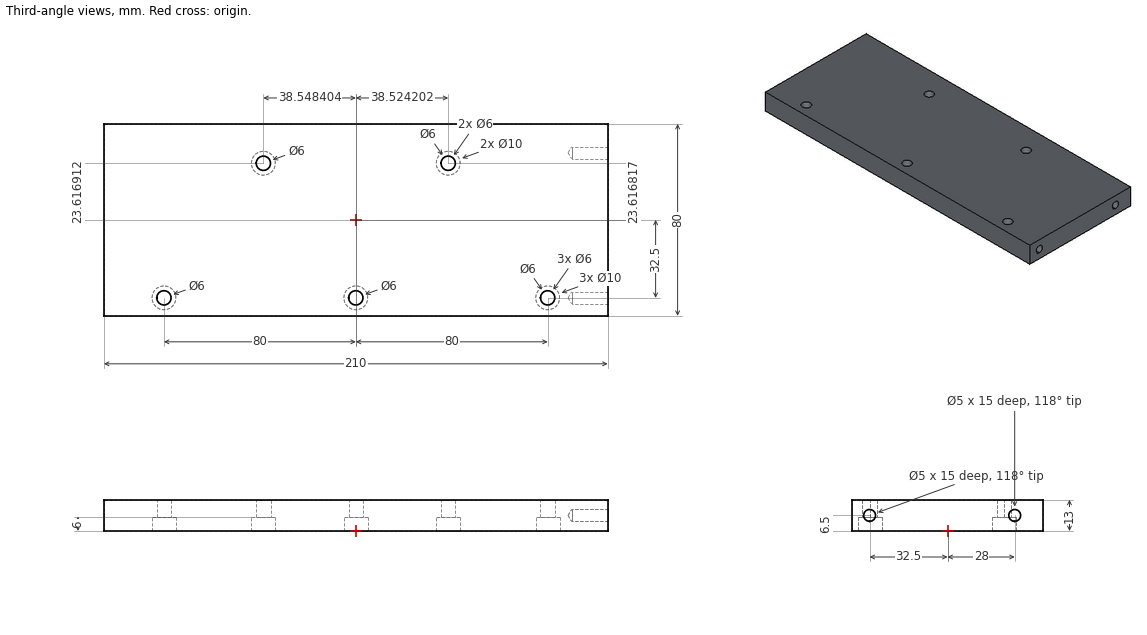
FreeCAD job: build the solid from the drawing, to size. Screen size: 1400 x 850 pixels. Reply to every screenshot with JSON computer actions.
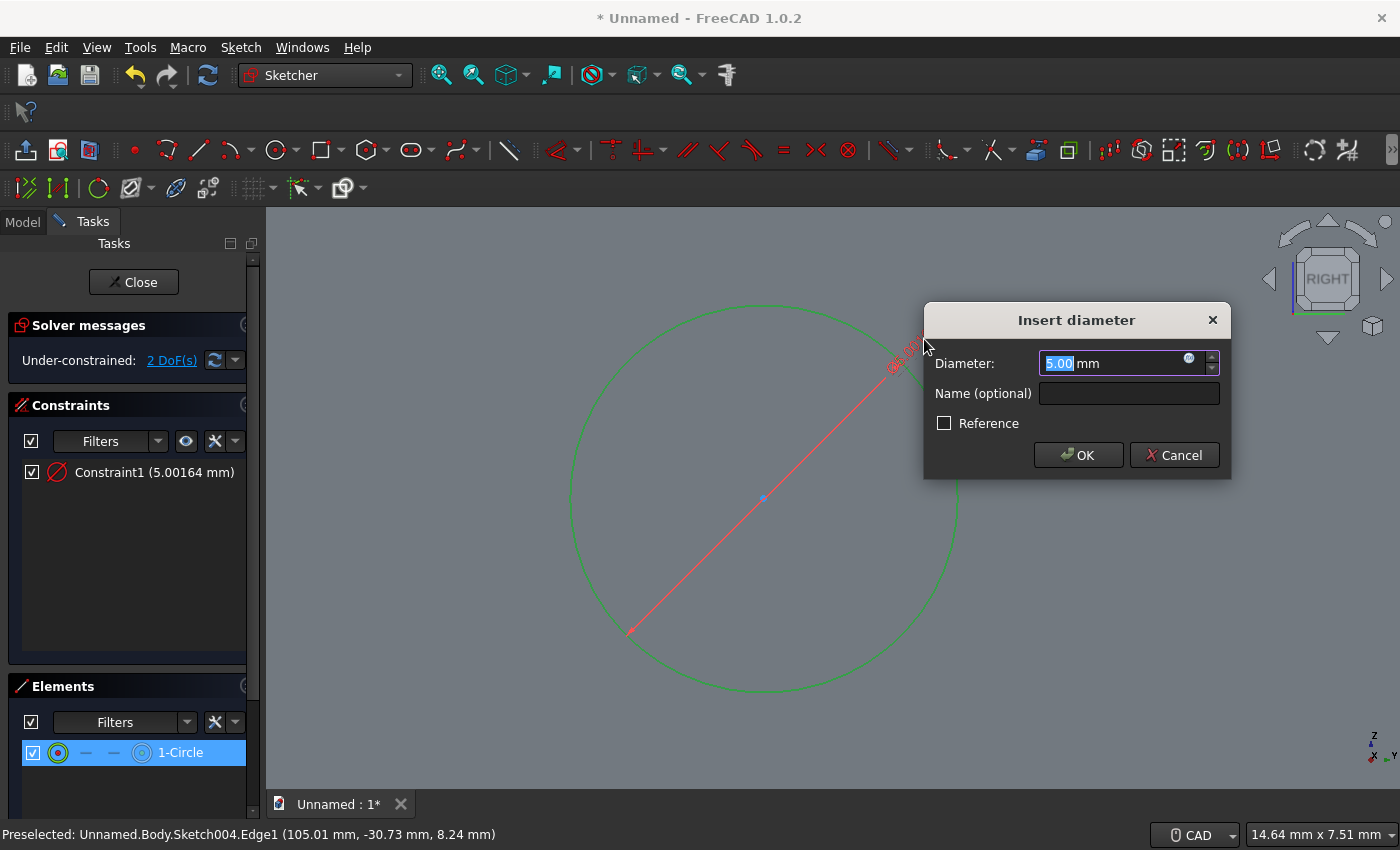
{"action": "type", "text": "5"}
{"action": "key", "text": "Return"}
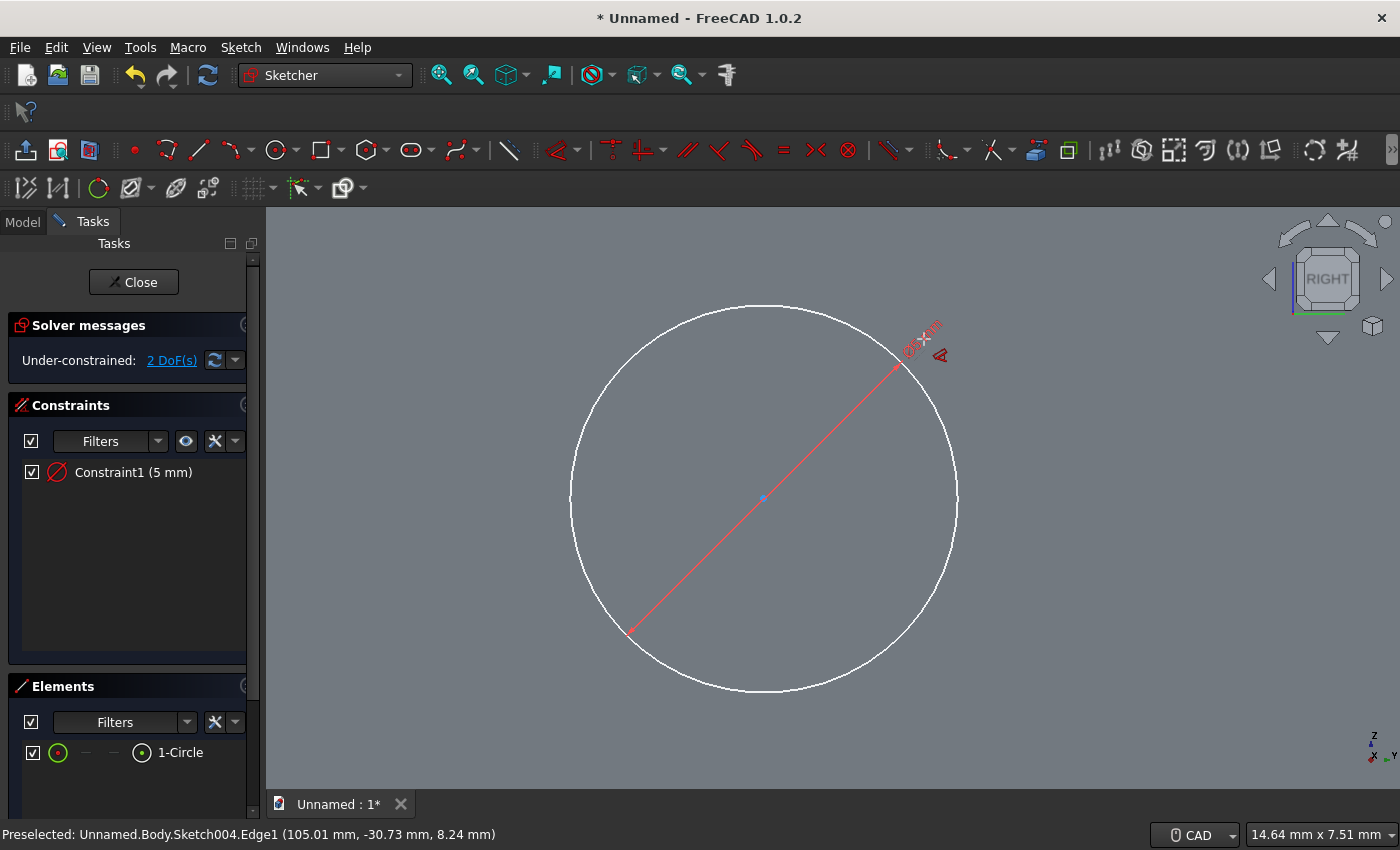
{"action": "left_click", "coordinate": [764, 499]}
{"action": "left_click", "coordinate": [730, 630]}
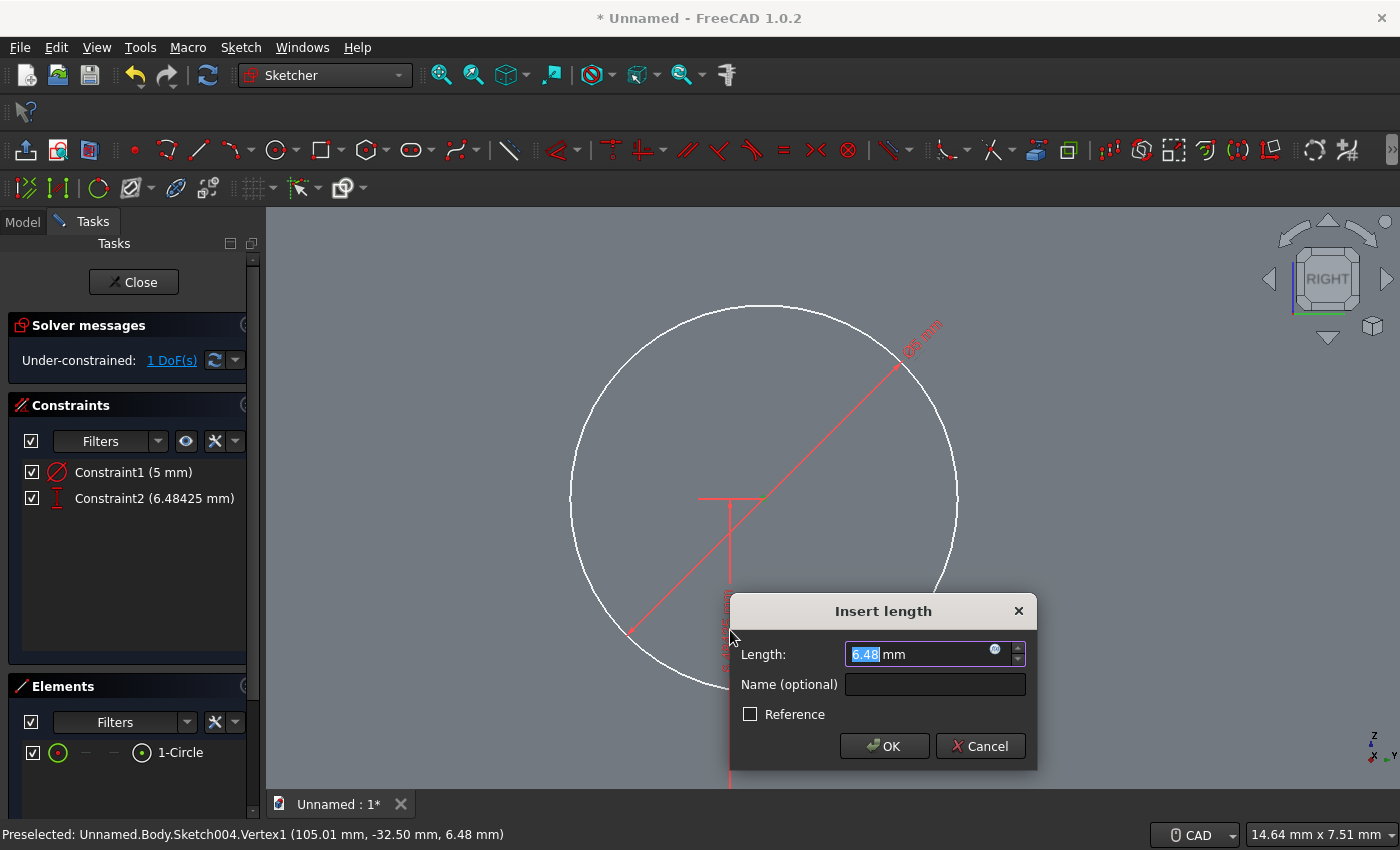
{"action": "type", "text": "6.5"}
{"action": "key", "text": "Return"}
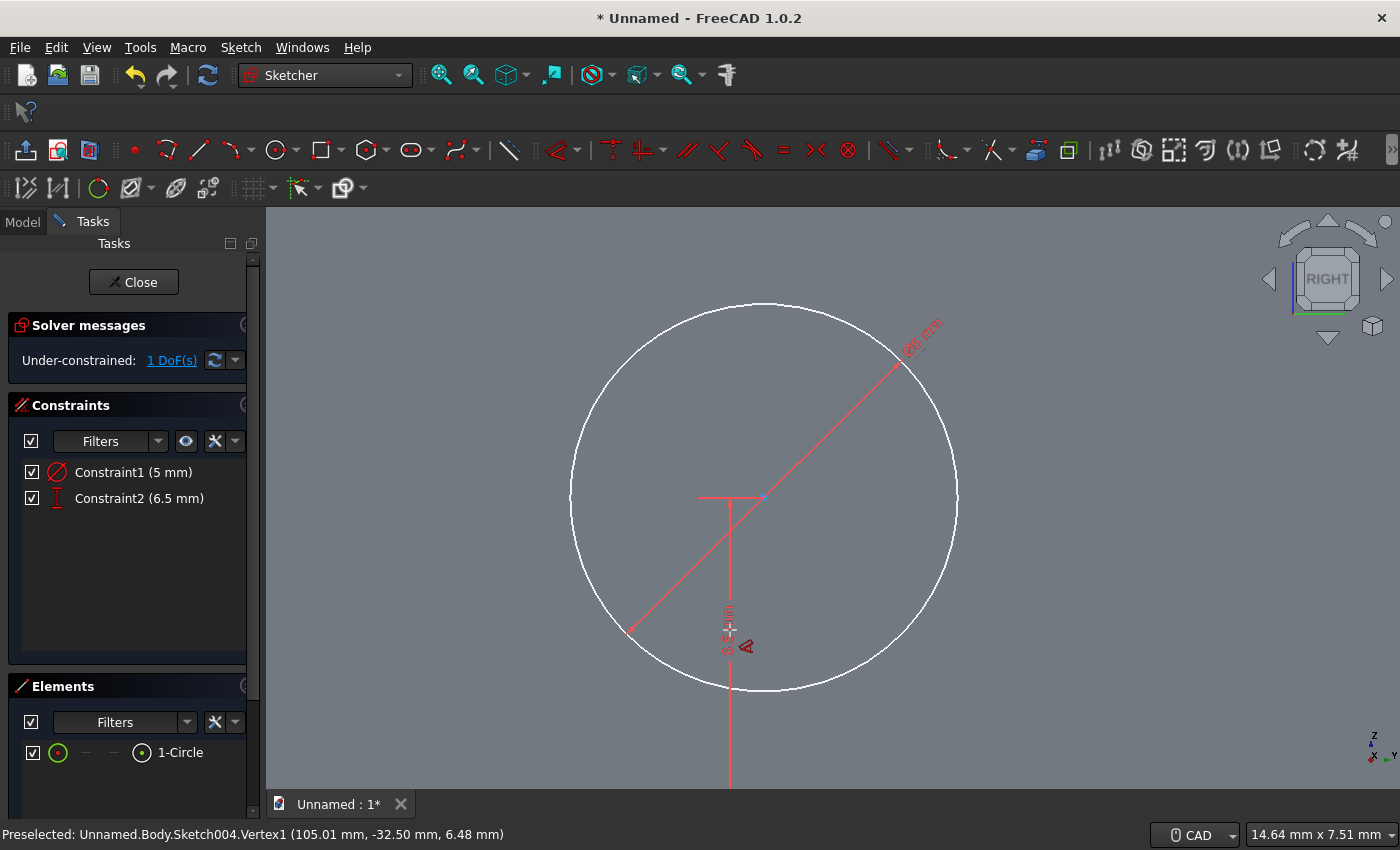
{"action": "left_click", "coordinate": [764, 498]}
{"action": "left_click", "coordinate": [999, 464]}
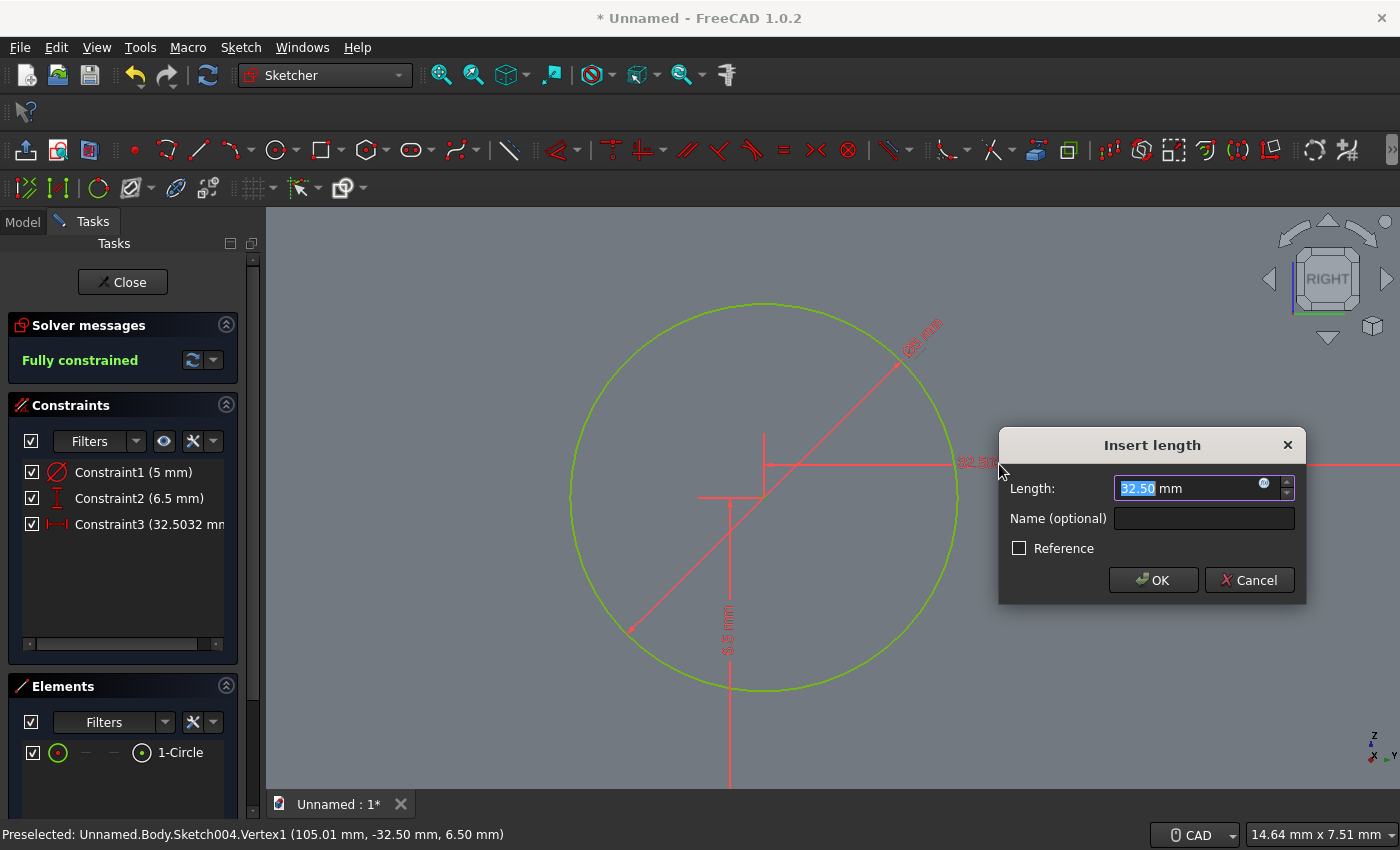
{"action": "type", "text": "32.5"}
{"action": "key", "text": "Return"}
{"action": "key", "text": "Escape"}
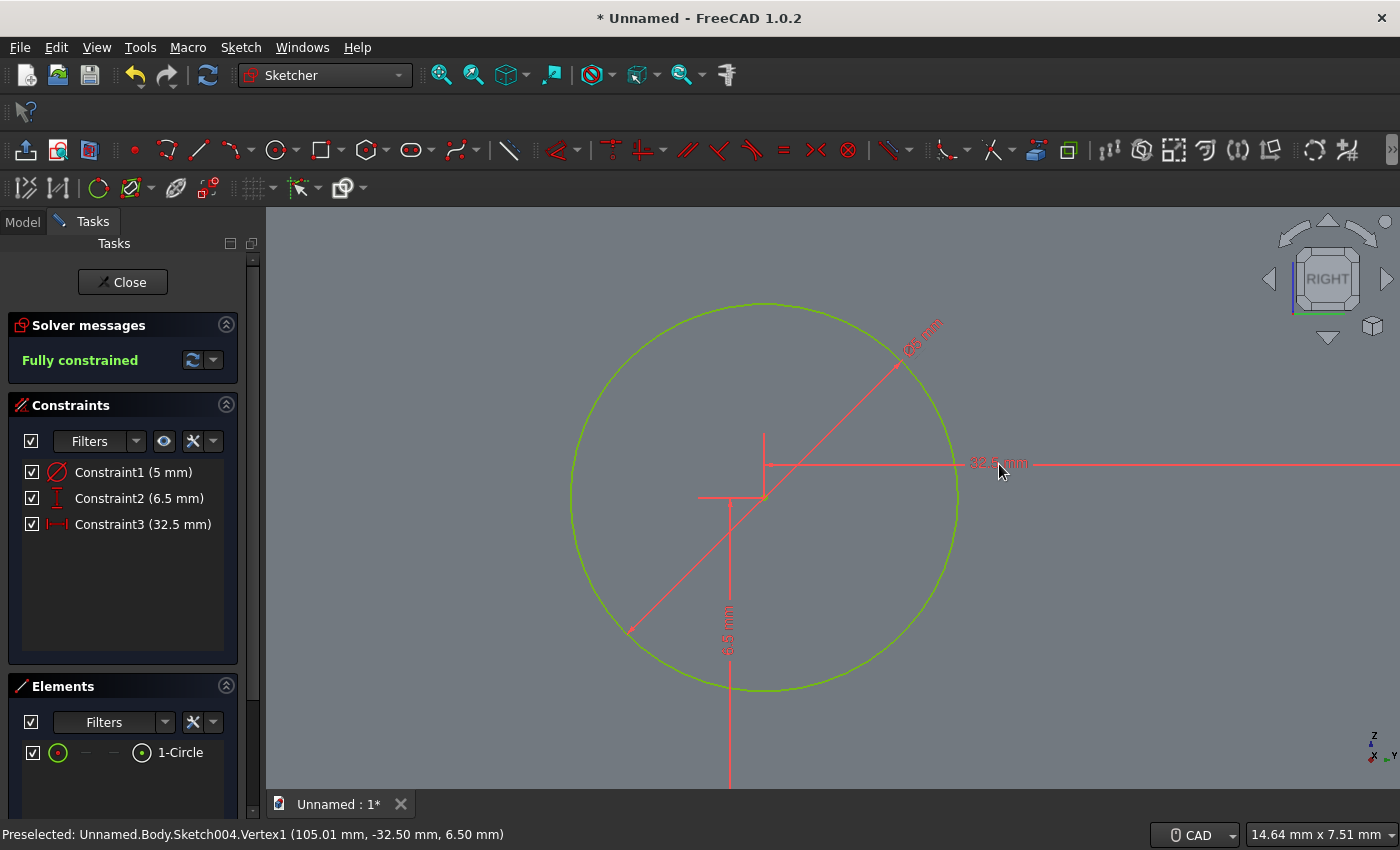
{"action": "left_click", "coordinate": [123, 282]}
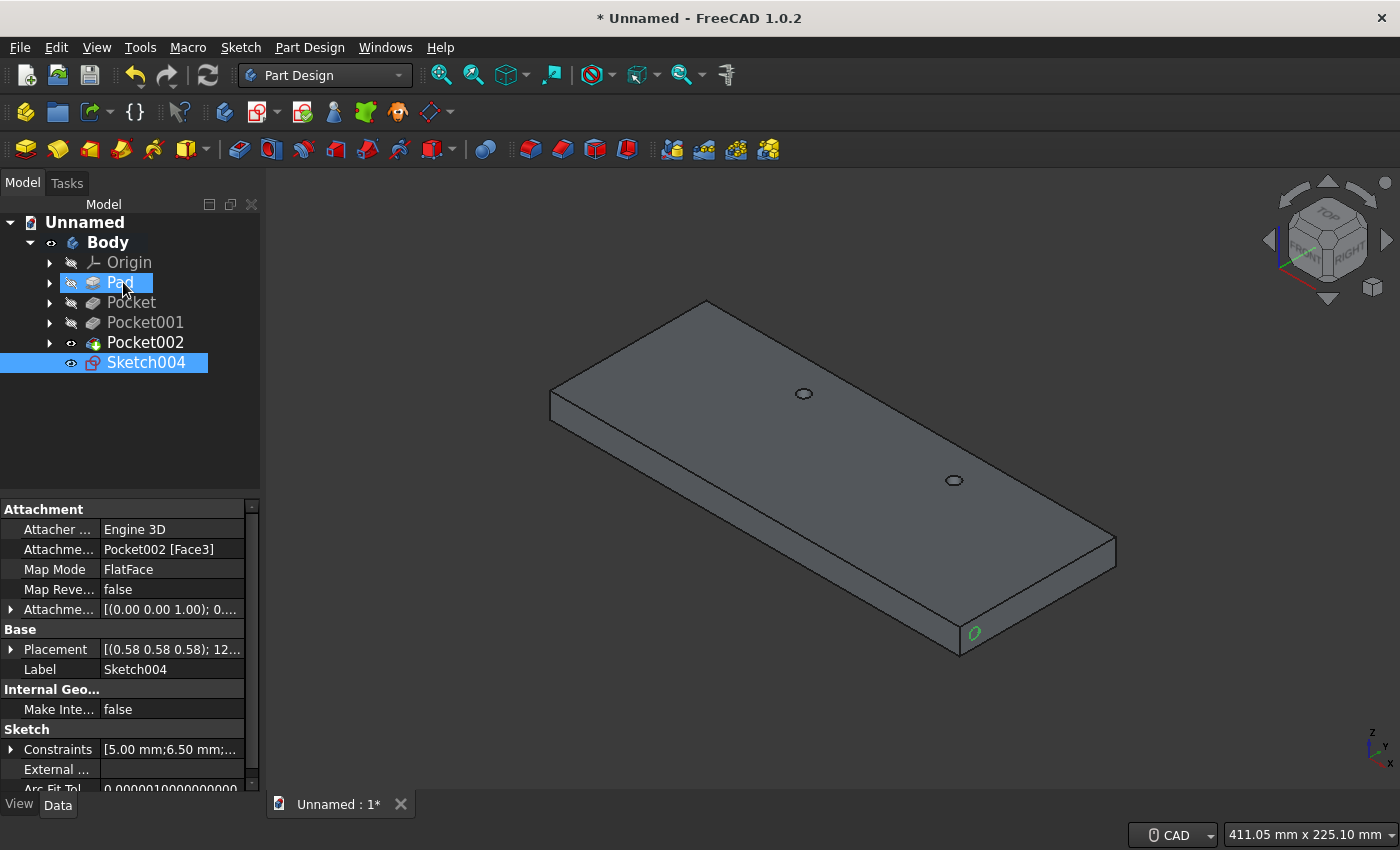
{"action": "left_click", "coordinate": [272, 150]}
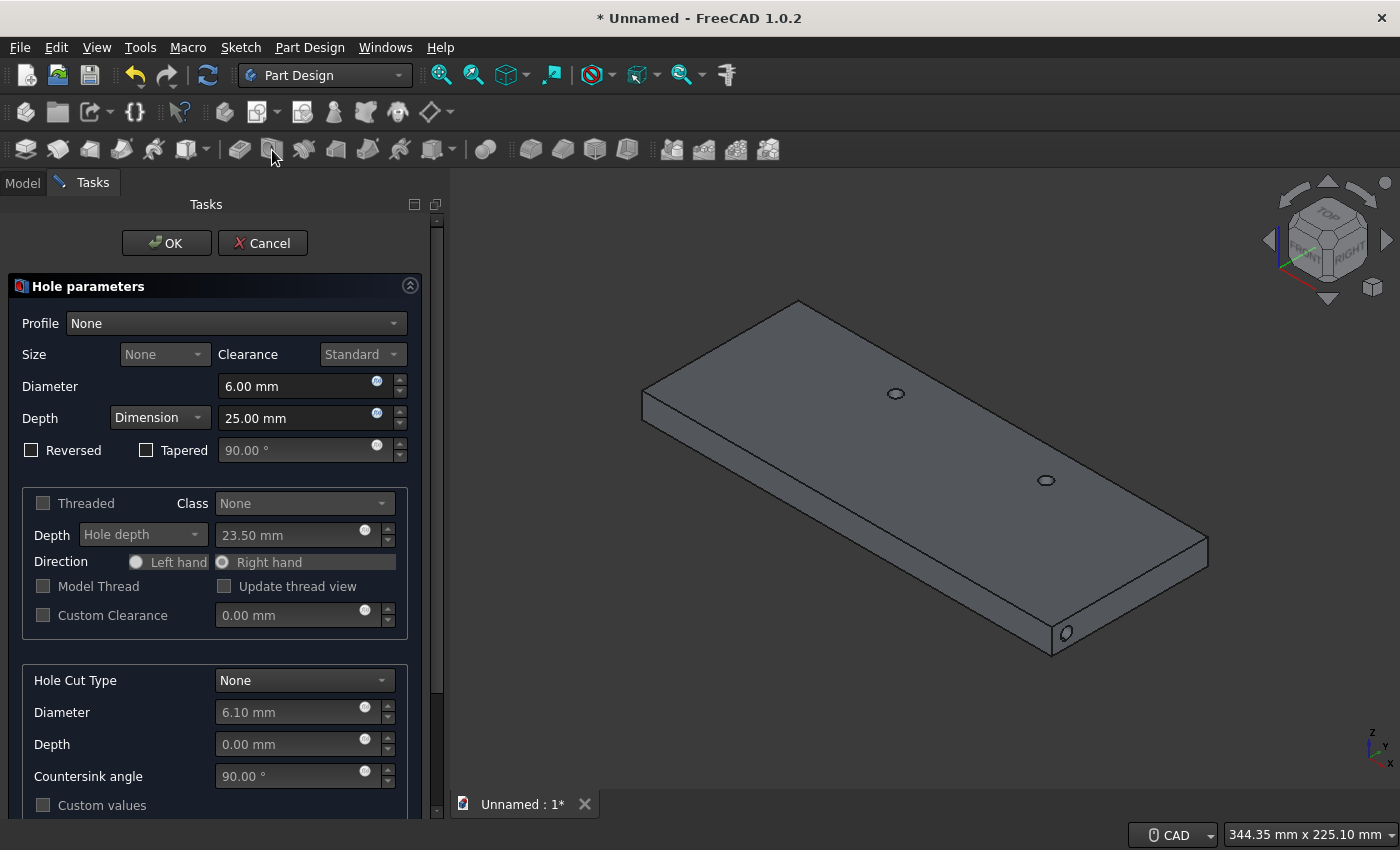
{"action": "triple_click", "coordinate": [305, 386]}